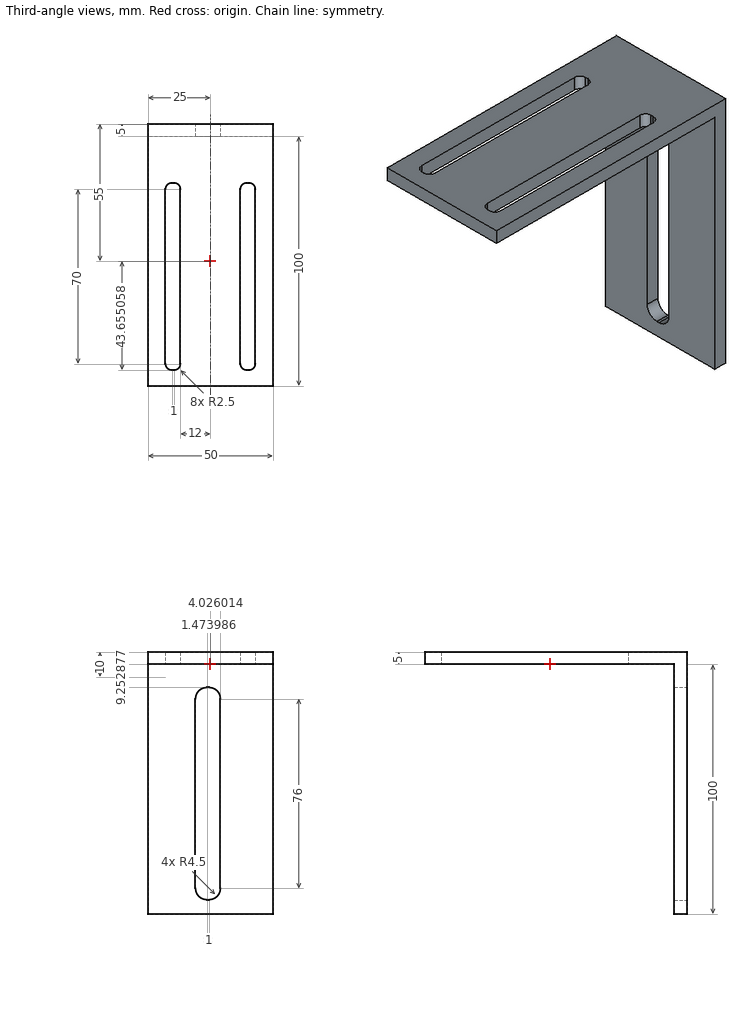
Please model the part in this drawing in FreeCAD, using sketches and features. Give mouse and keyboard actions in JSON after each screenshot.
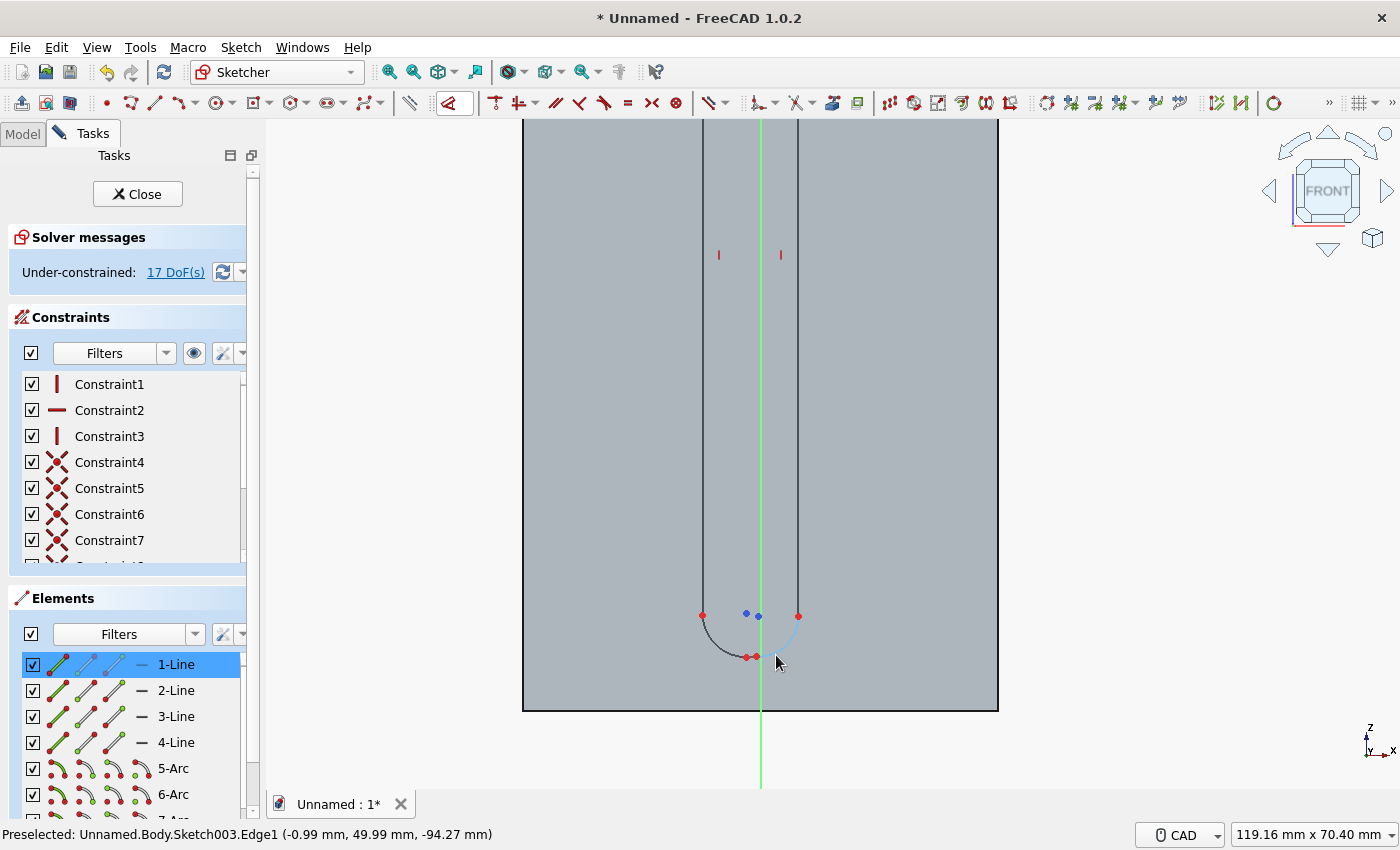
{"action": "left_click", "coordinate": [775, 653]}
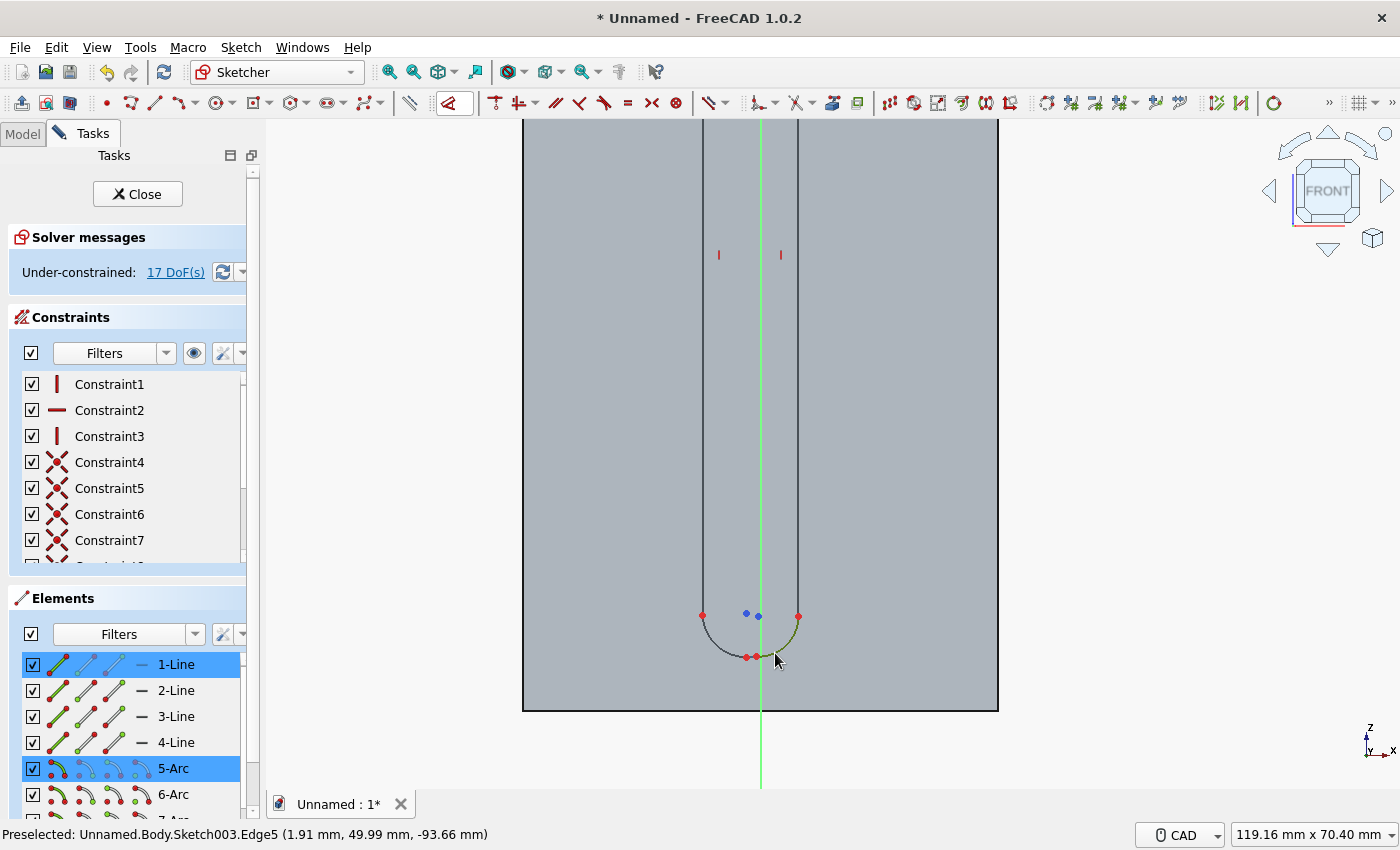
{"action": "left_click", "coordinate": [604, 104]}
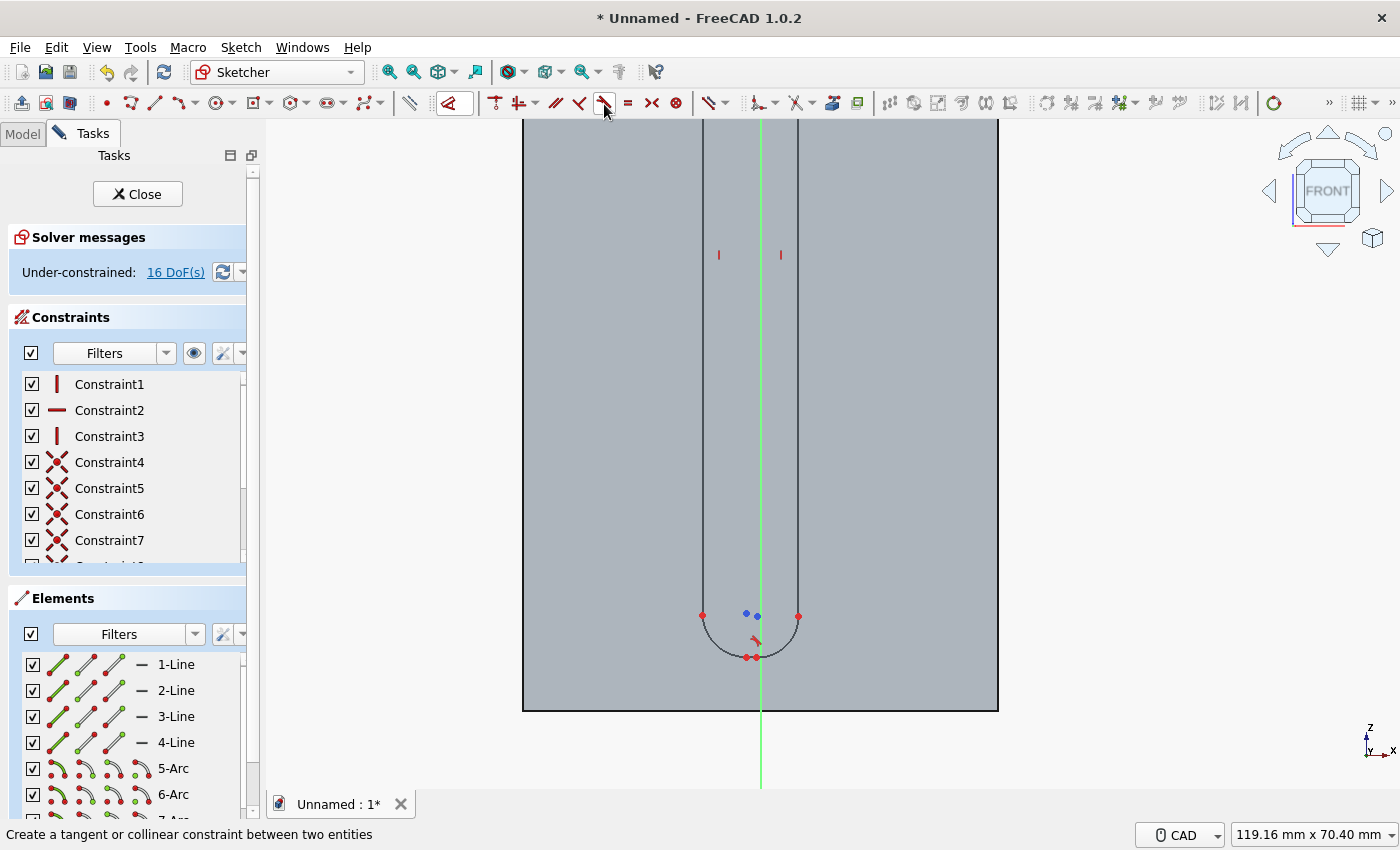
{"action": "scroll", "coordinate": [751, 657], "scroll_direction": "up", "scroll_amount": 6}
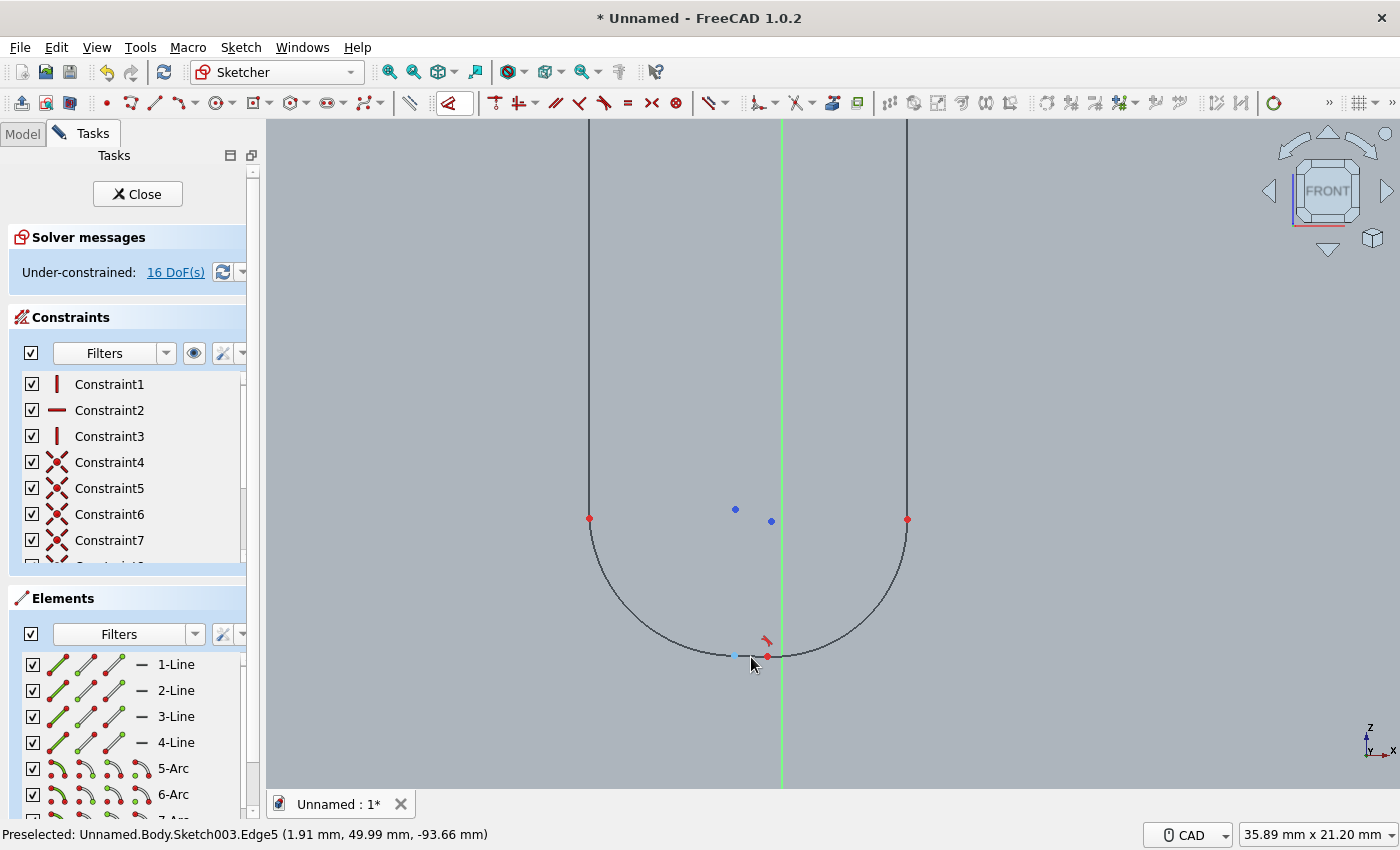
{"action": "left_click", "coordinate": [751, 656]}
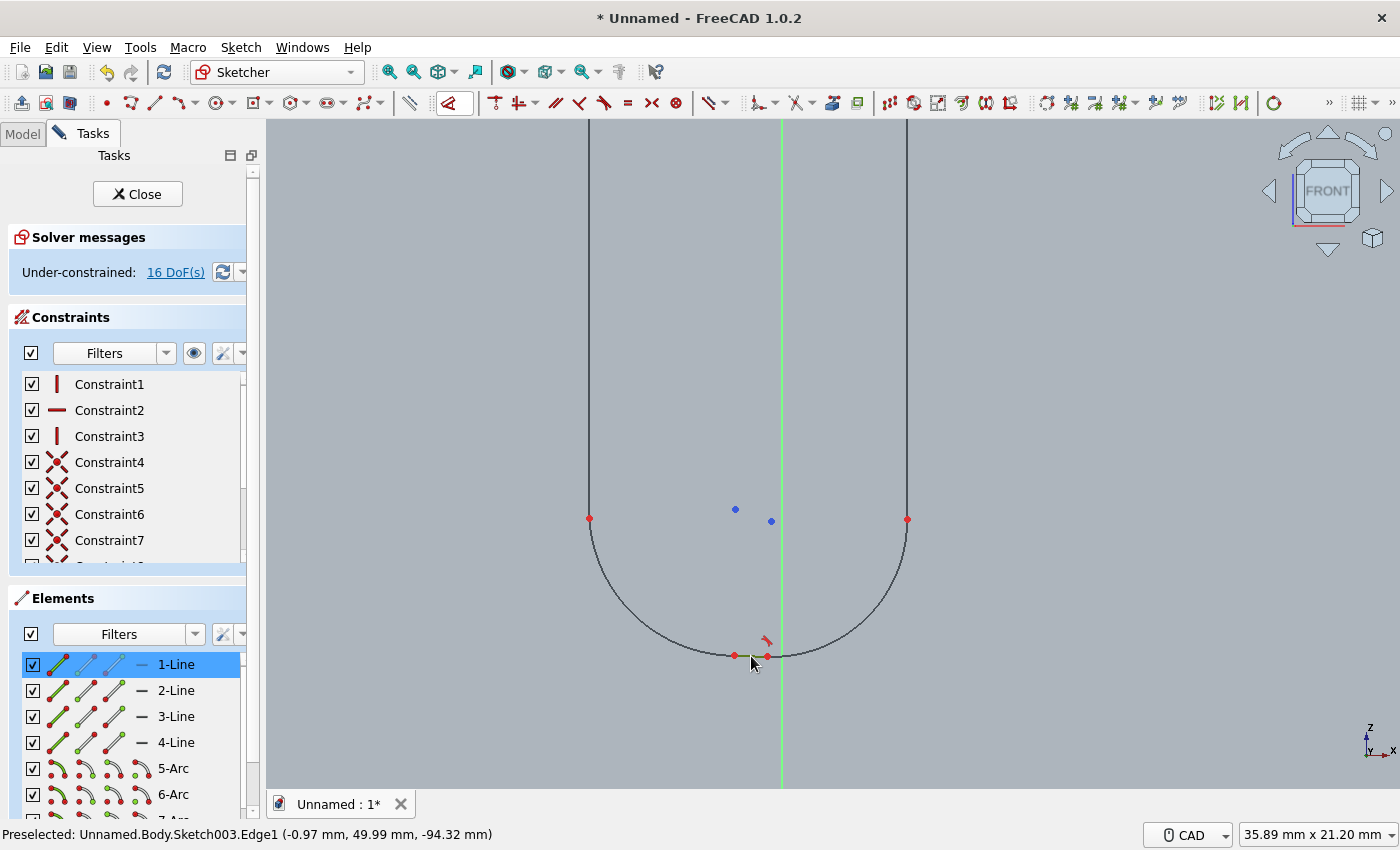
{"action": "scroll", "coordinate": [767, 656], "scroll_direction": "down", "scroll_amount": 10}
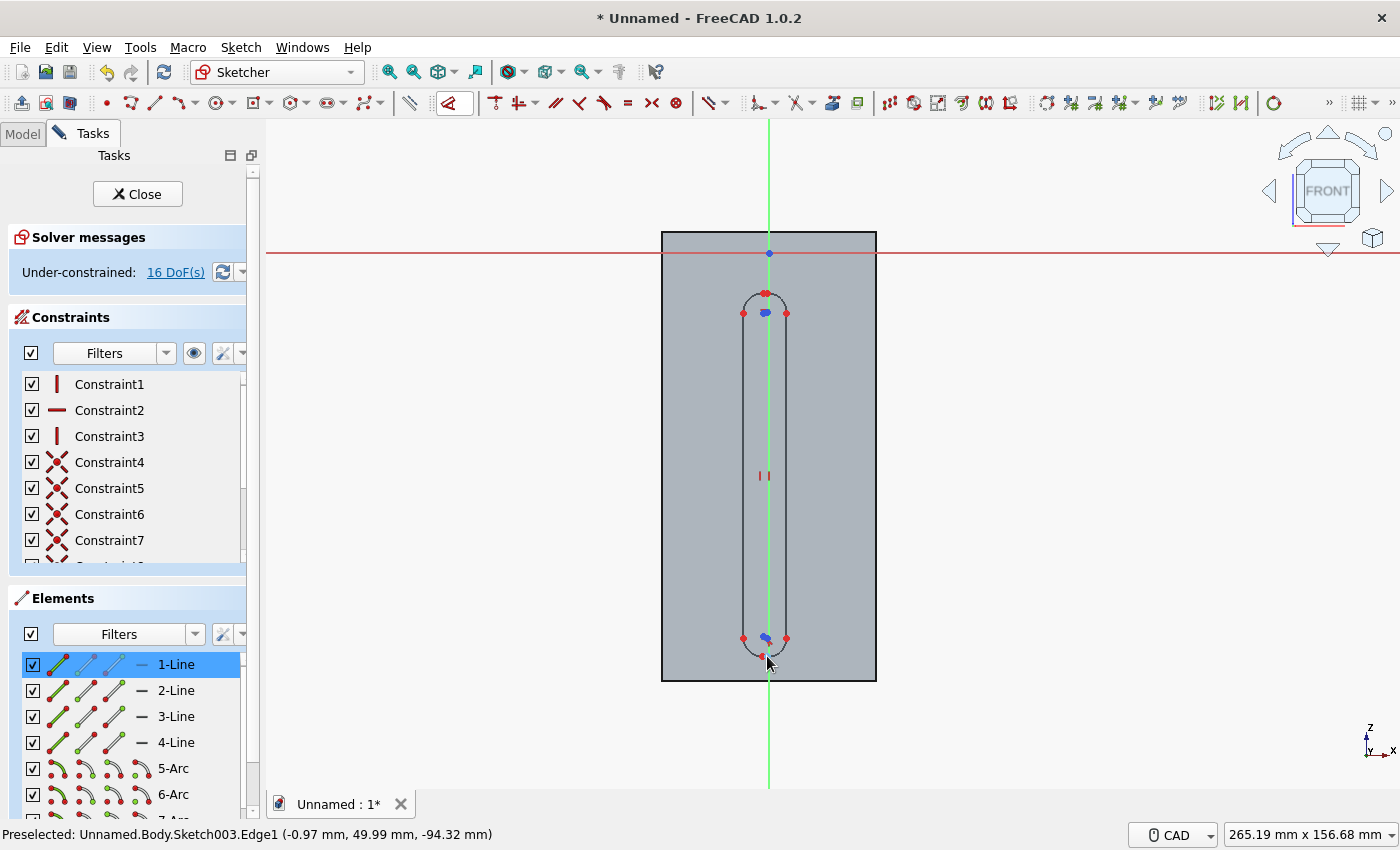
{"action": "scroll", "coordinate": [746, 647], "scroll_direction": "up", "scroll_amount": 3}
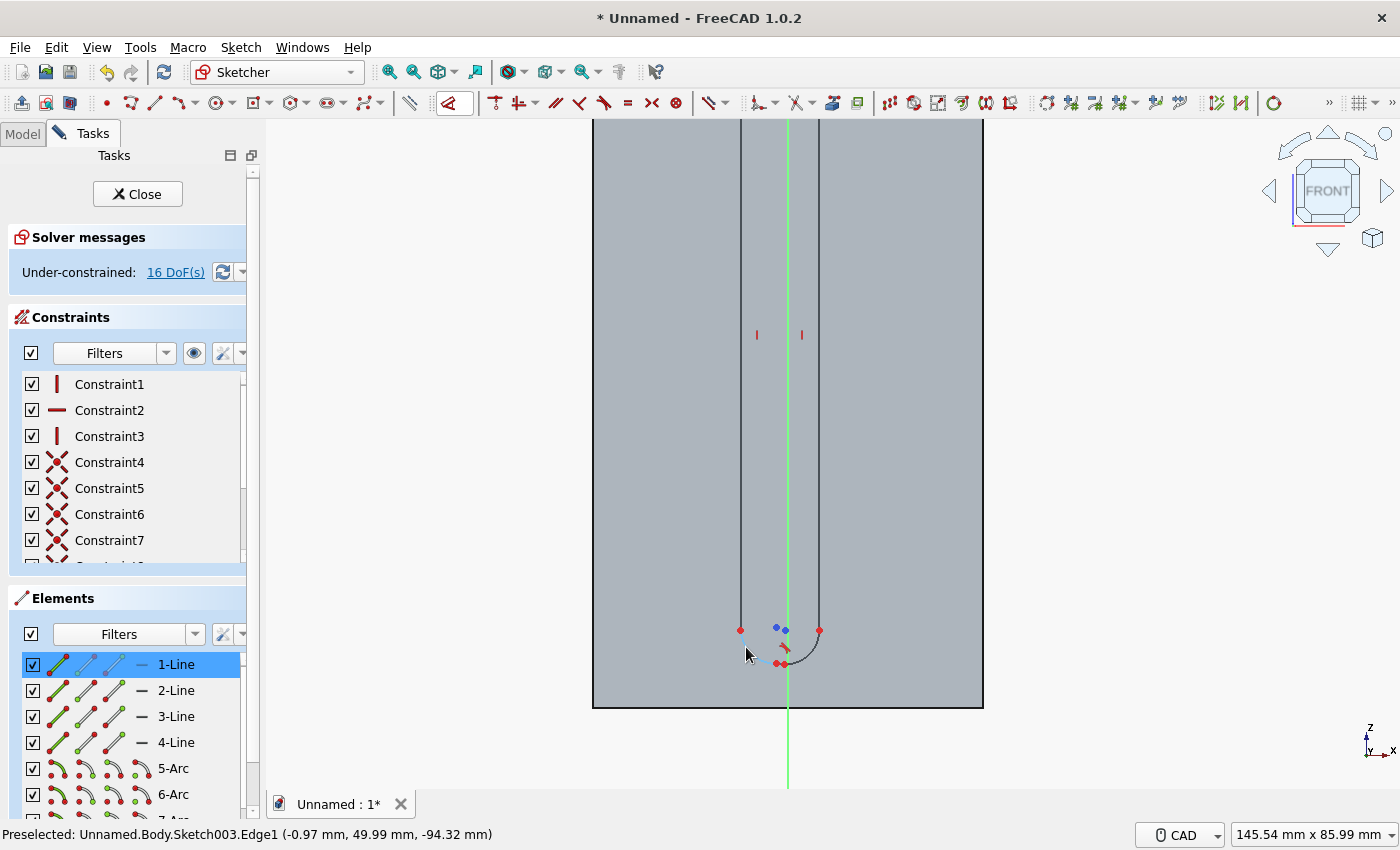
{"action": "left_click", "coordinate": [745, 646]}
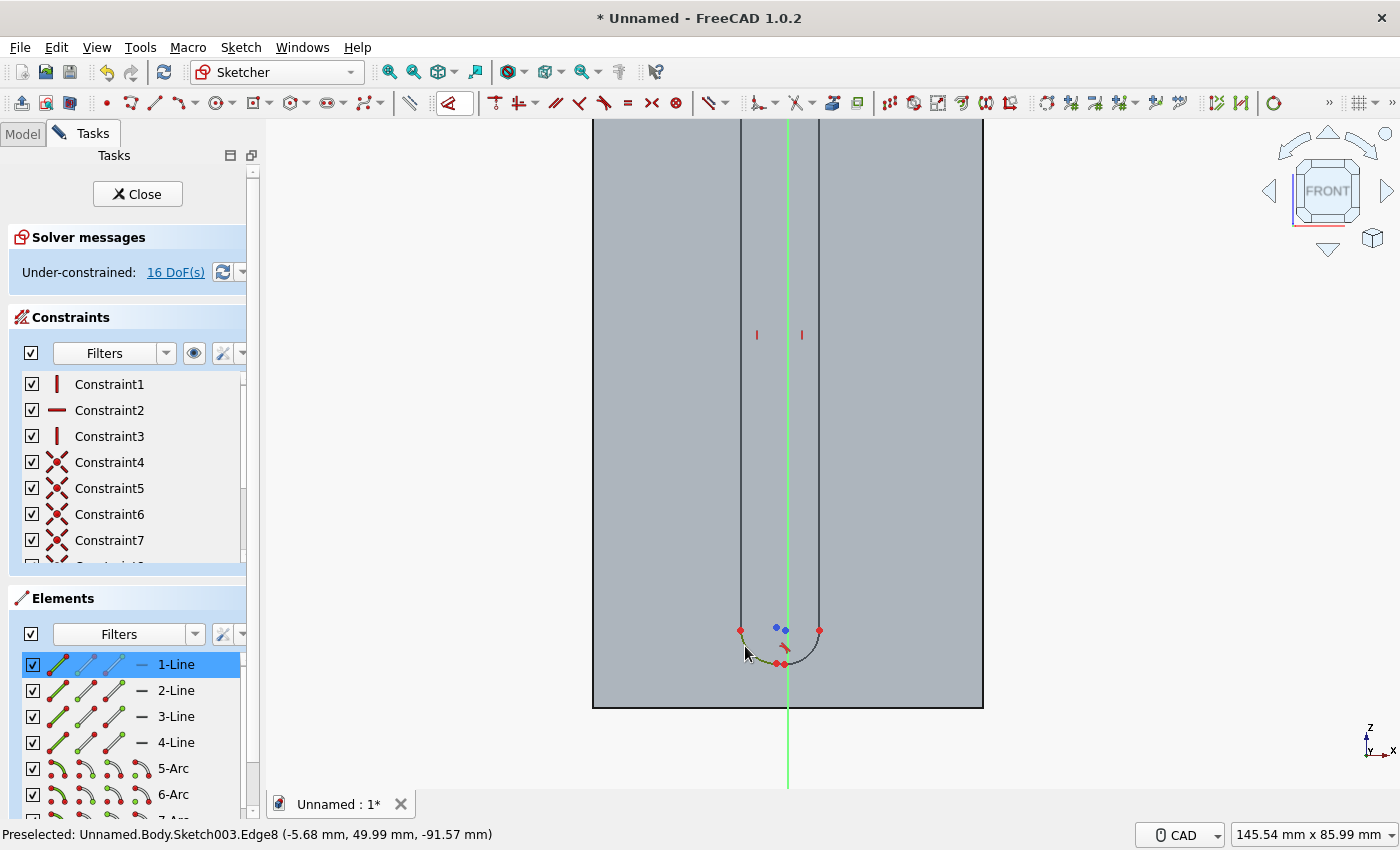
{"action": "key", "text": "t"}